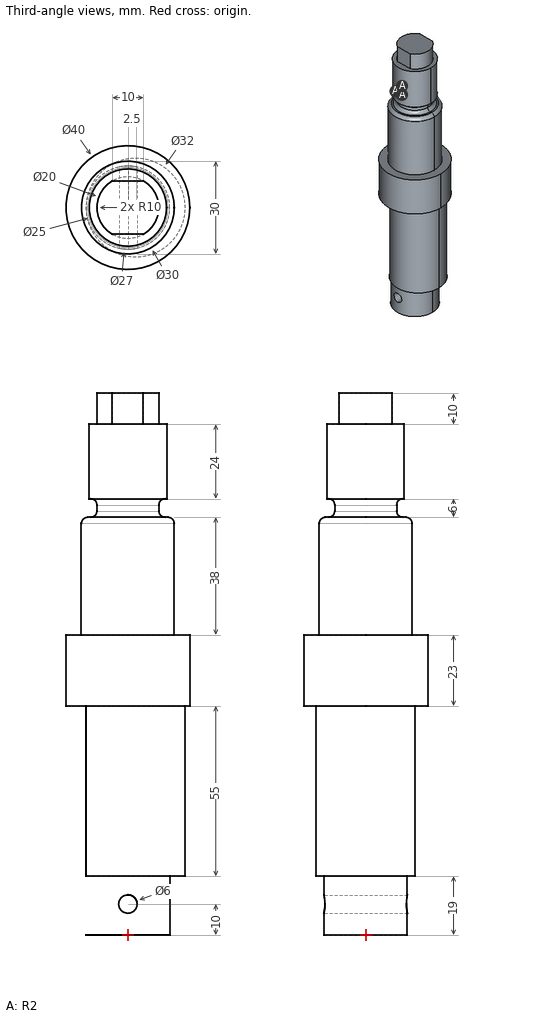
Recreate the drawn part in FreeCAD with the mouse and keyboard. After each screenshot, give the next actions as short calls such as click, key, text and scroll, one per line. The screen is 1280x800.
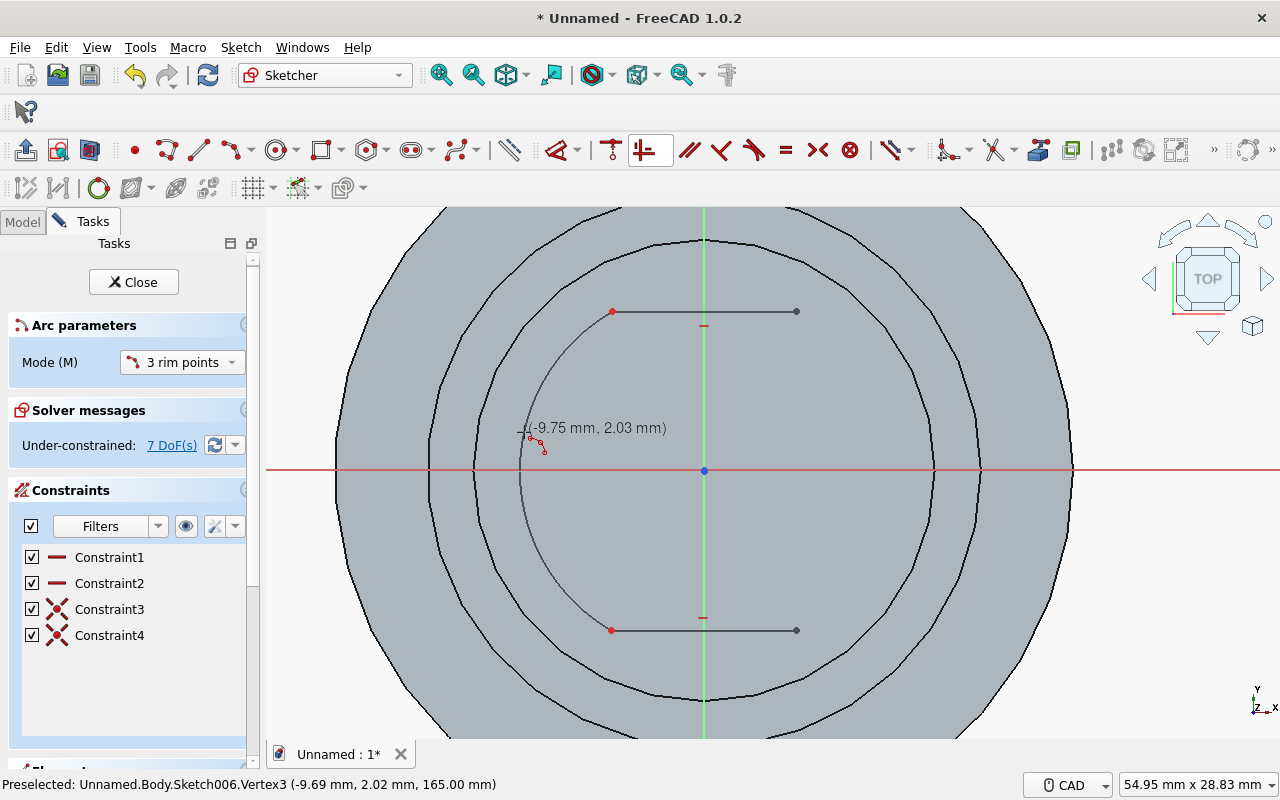
click(796, 631)
click(796, 312)
click(885, 509)
key(Escape)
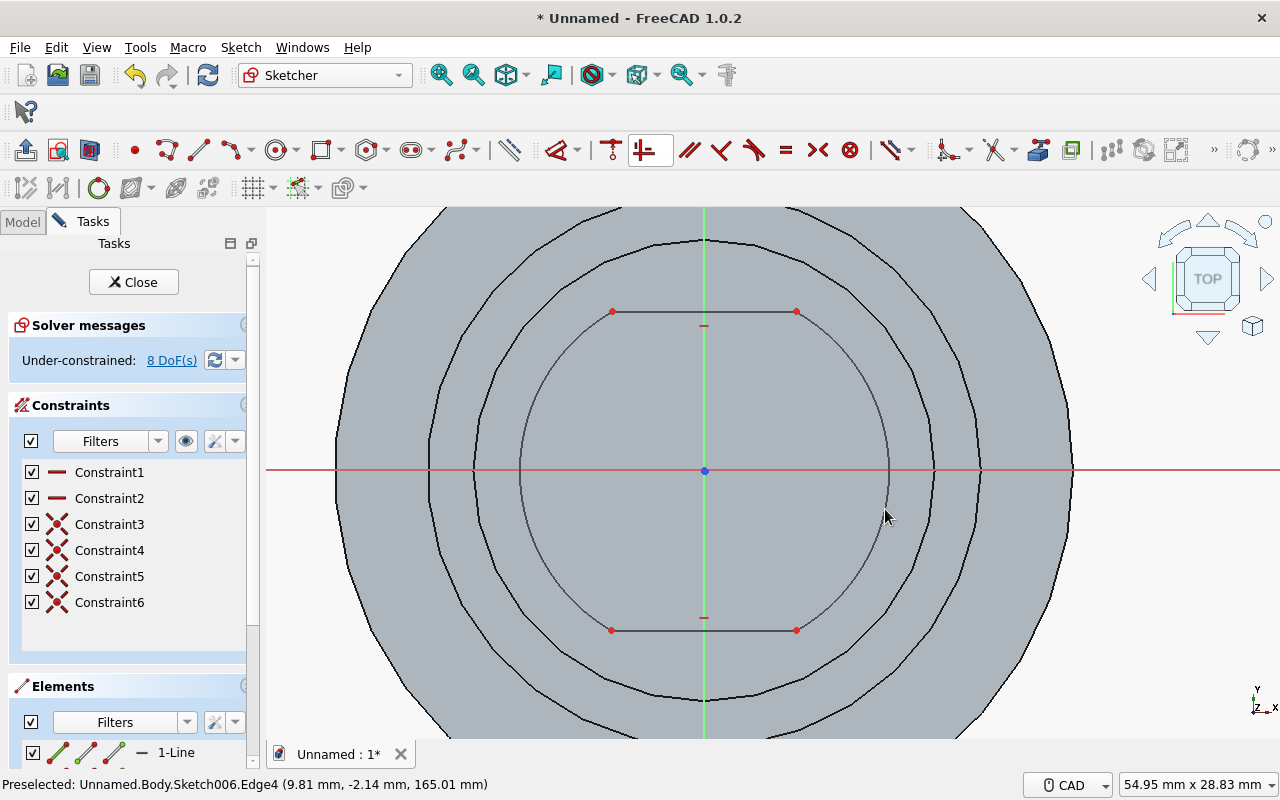
click(536, 397)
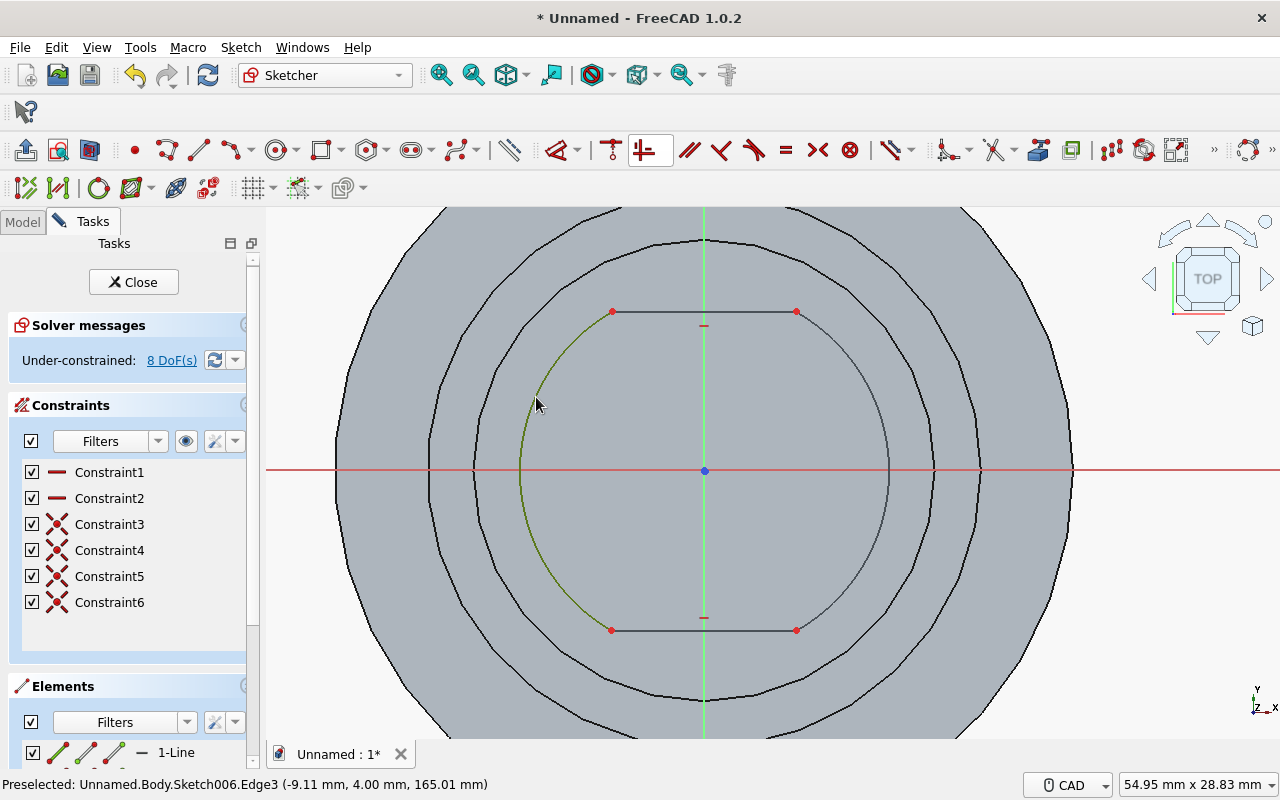
click(873, 547)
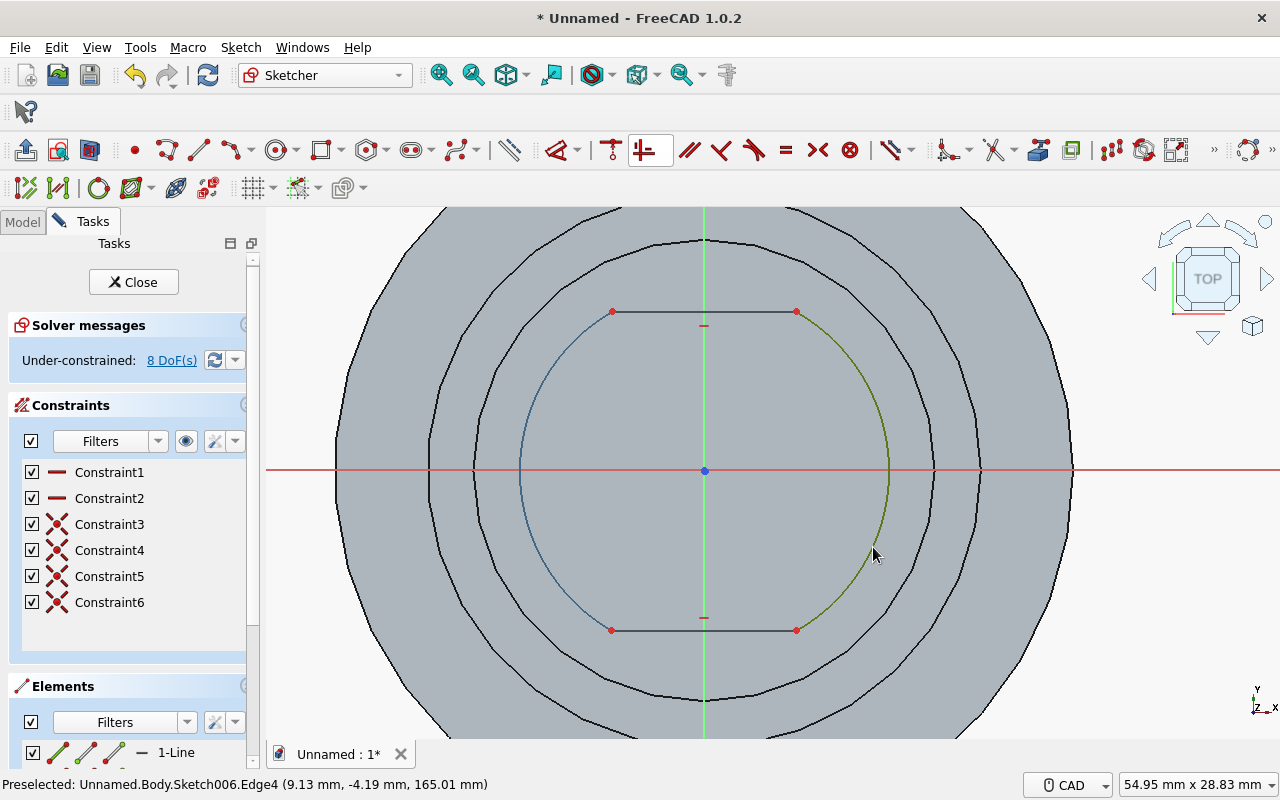
key(c)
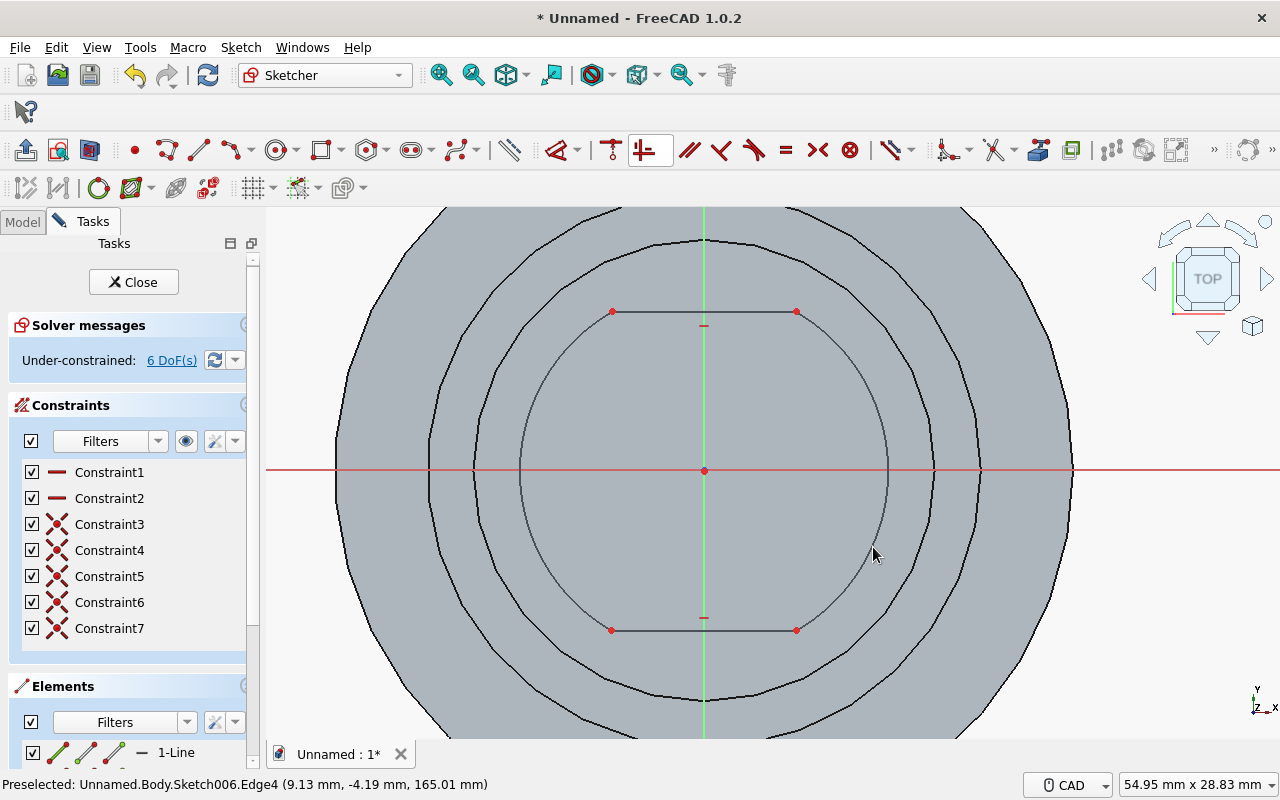
drag(694, 460, 714, 481)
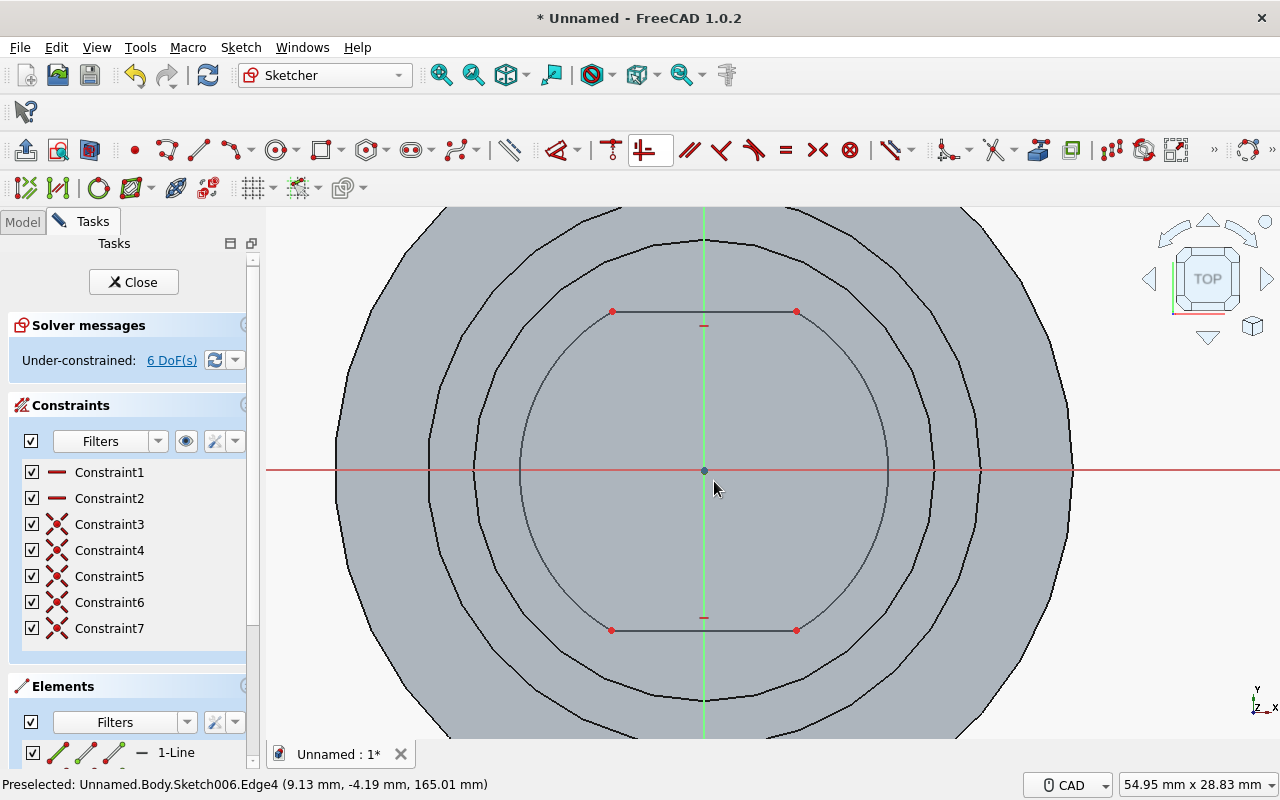
click(612, 150)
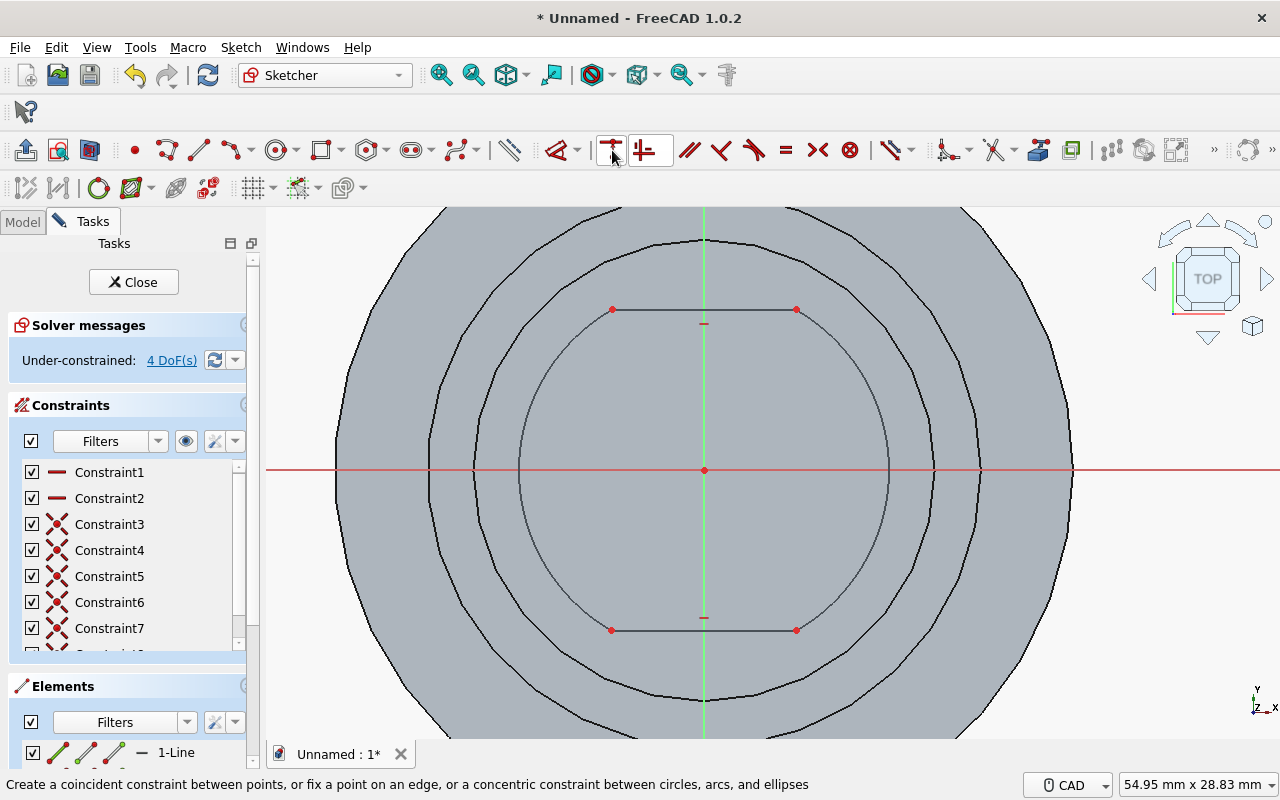
click(535, 395)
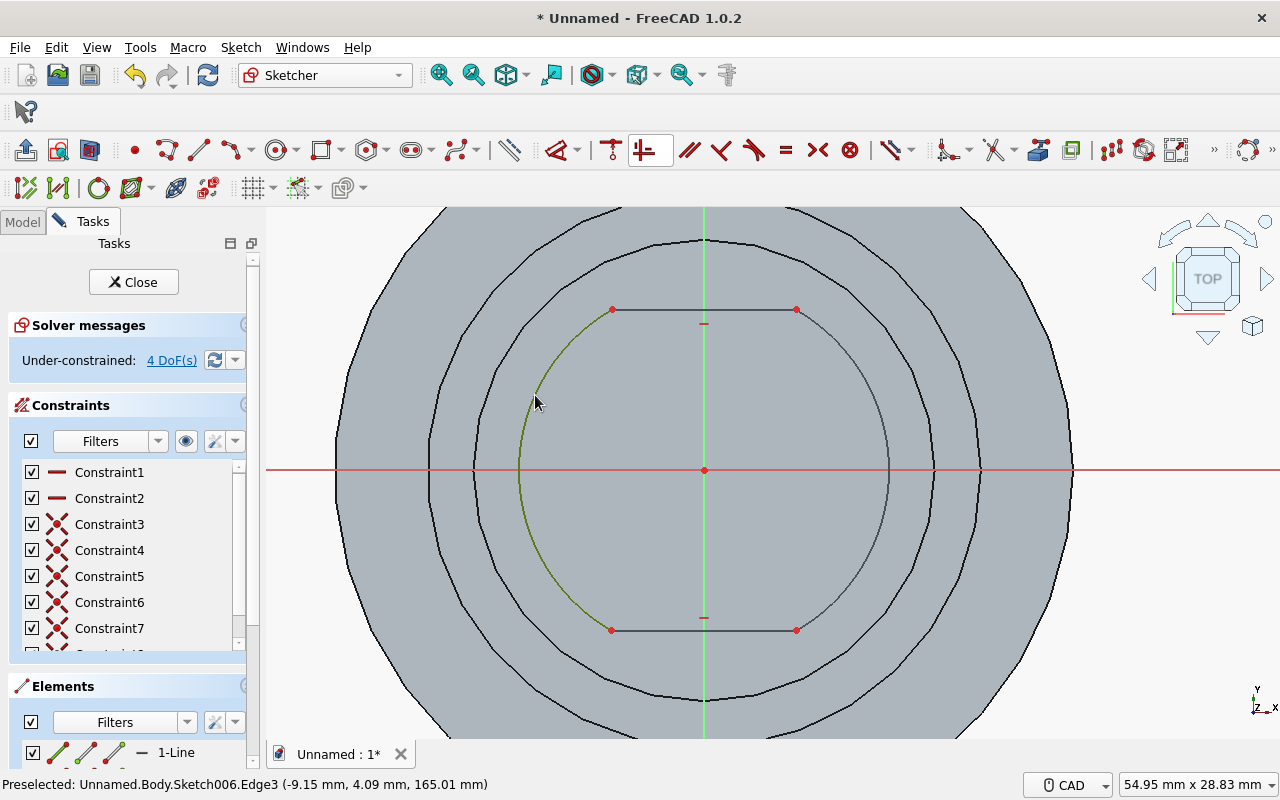
click(873, 546)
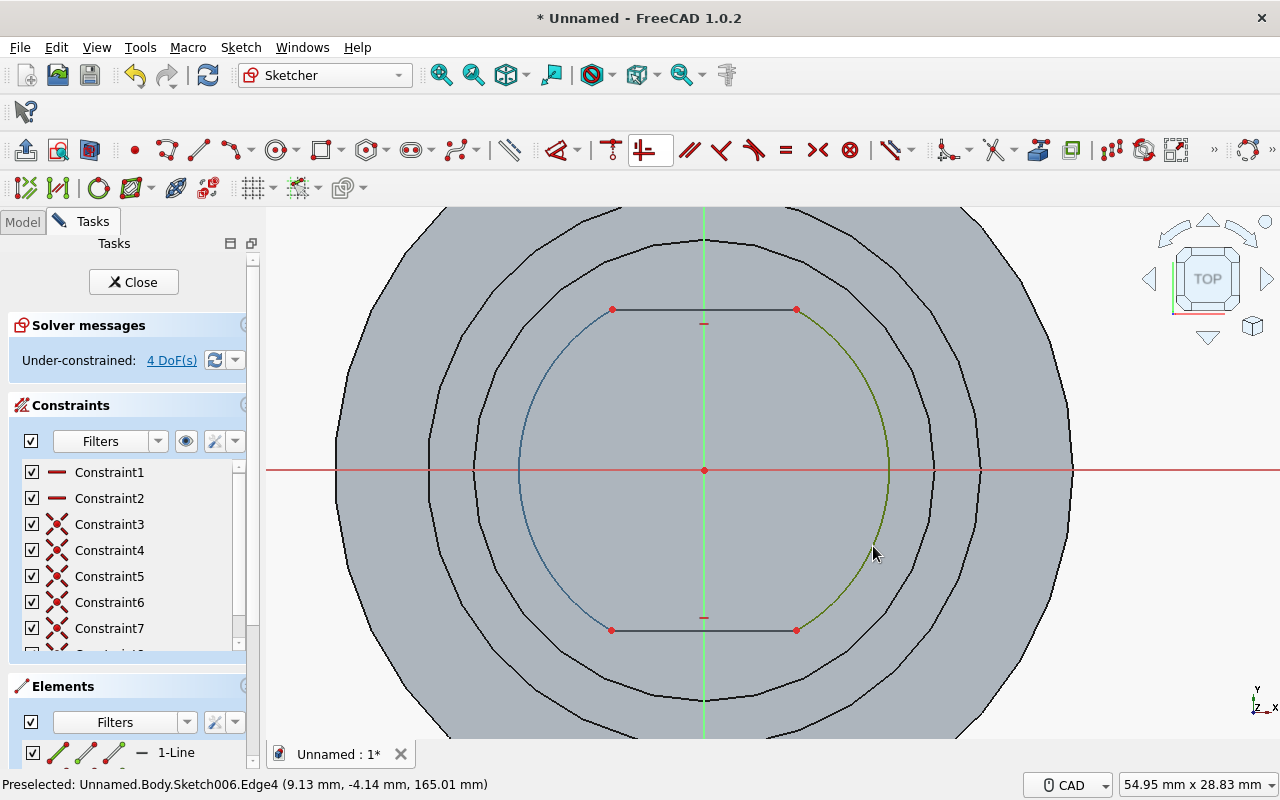
key(e)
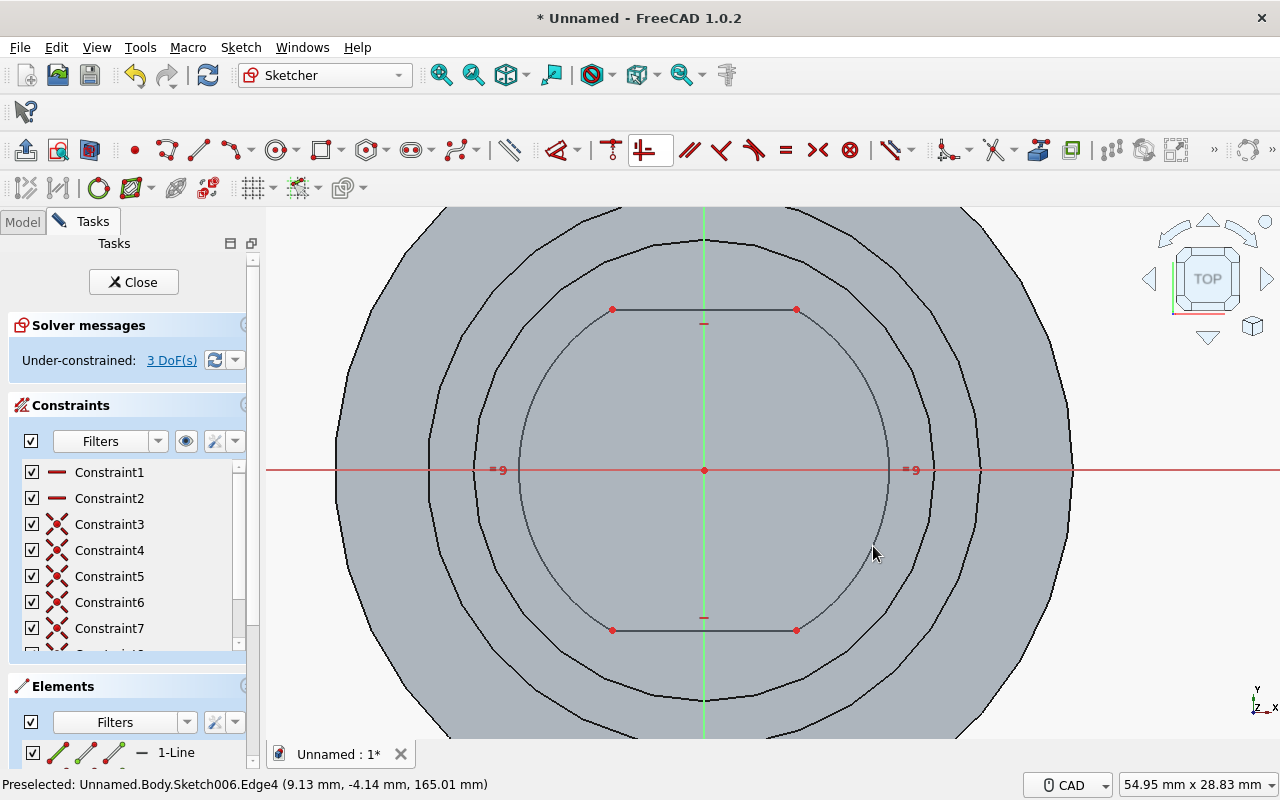
click(556, 150)